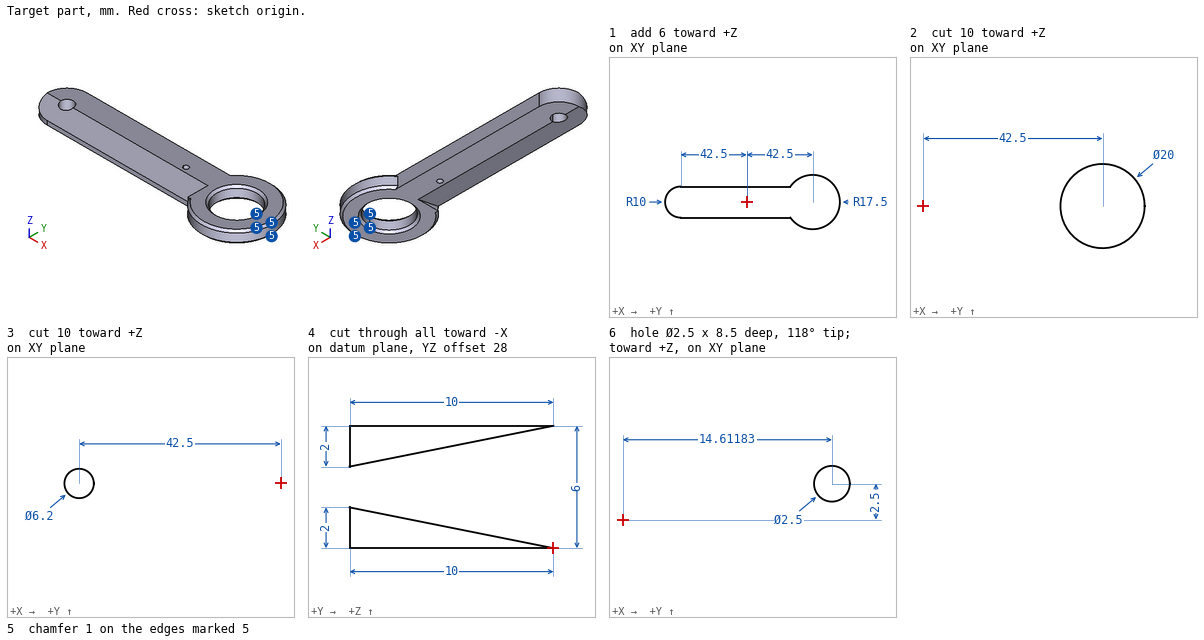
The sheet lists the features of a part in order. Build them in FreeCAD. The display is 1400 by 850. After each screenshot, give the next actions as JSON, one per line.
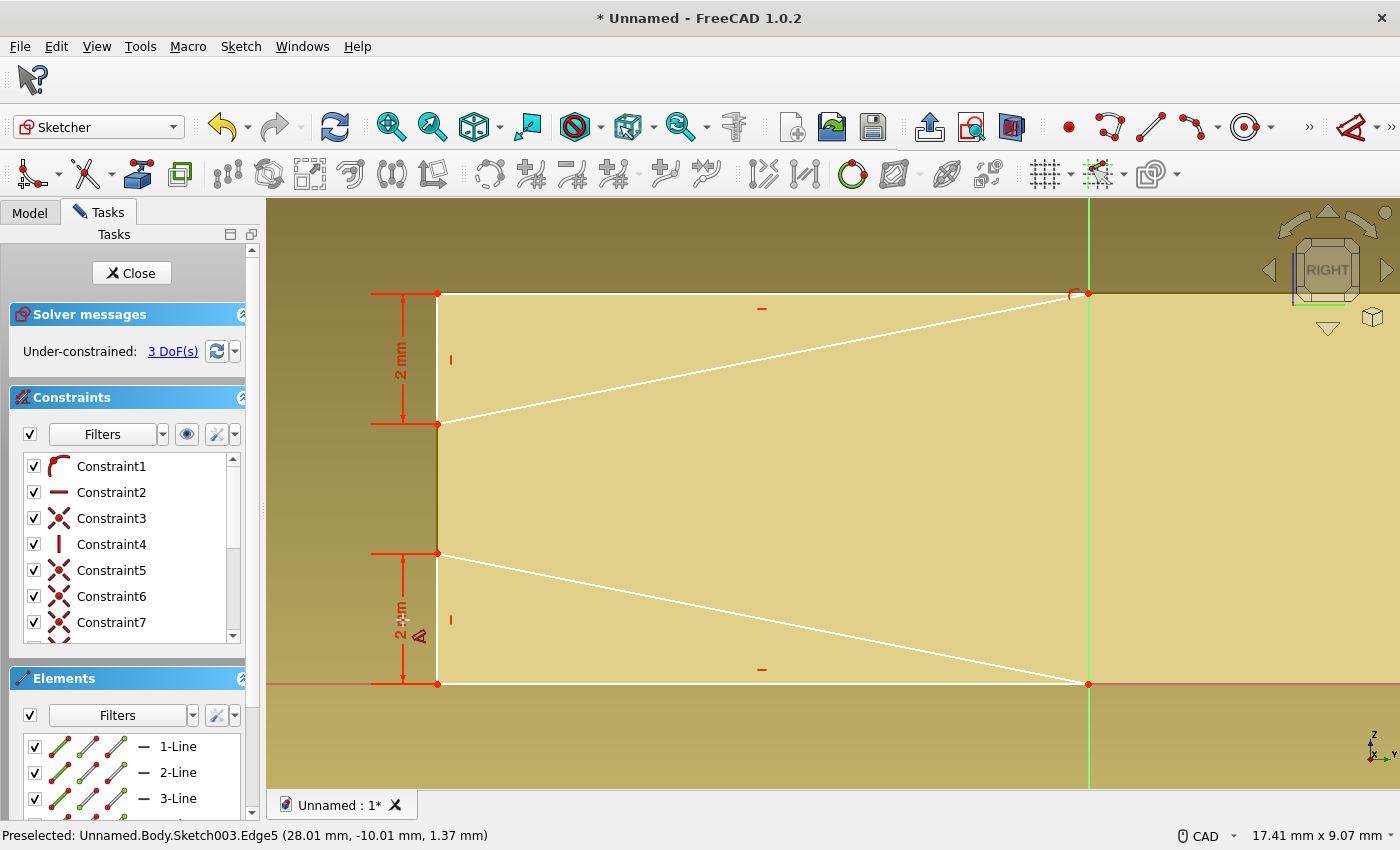
{"action": "left_click", "coordinate": [893, 294]}
{"action": "left_click", "coordinate": [763, 260]}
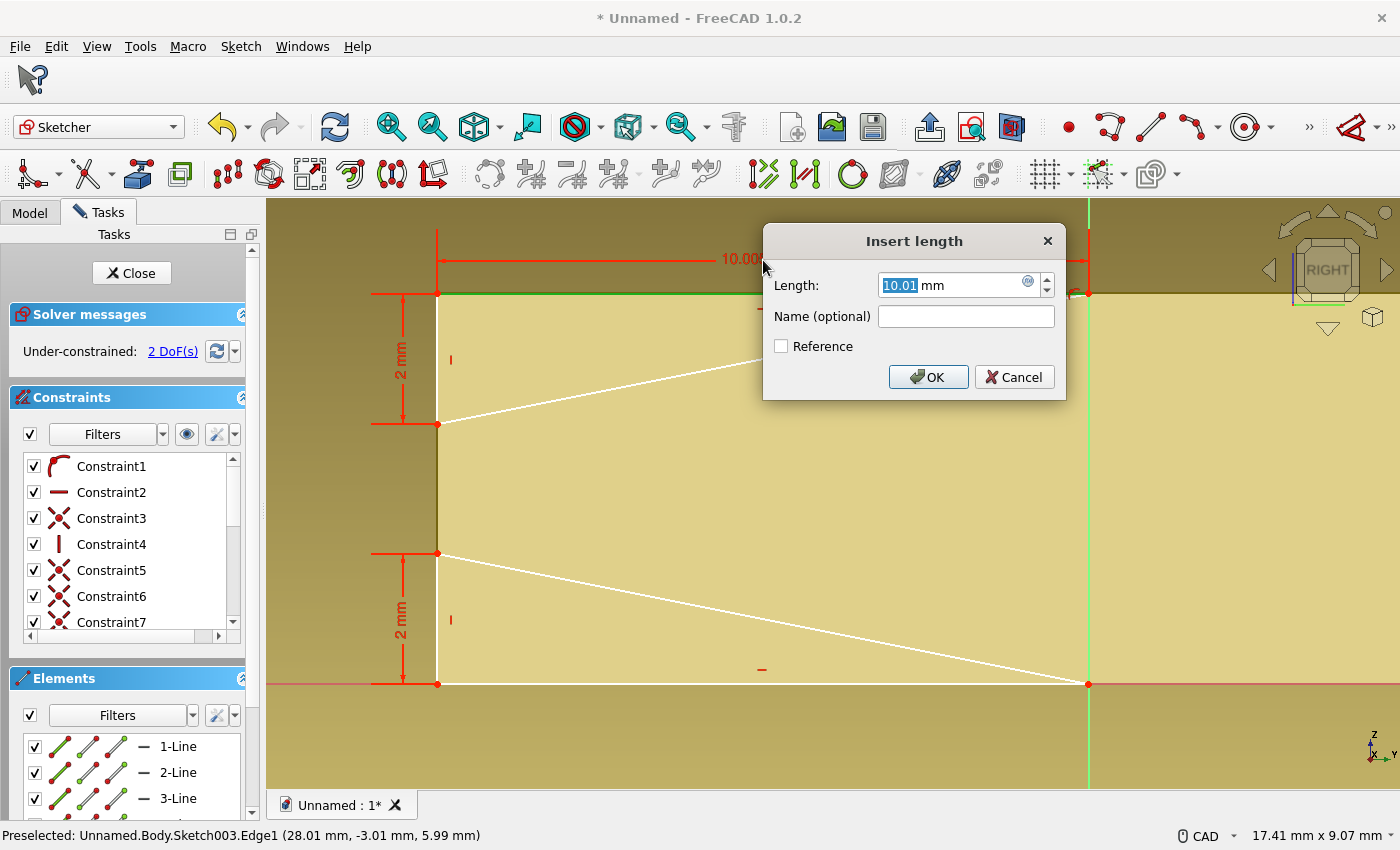
{"action": "type", "text": "10"}
{"action": "key", "text": "Return"}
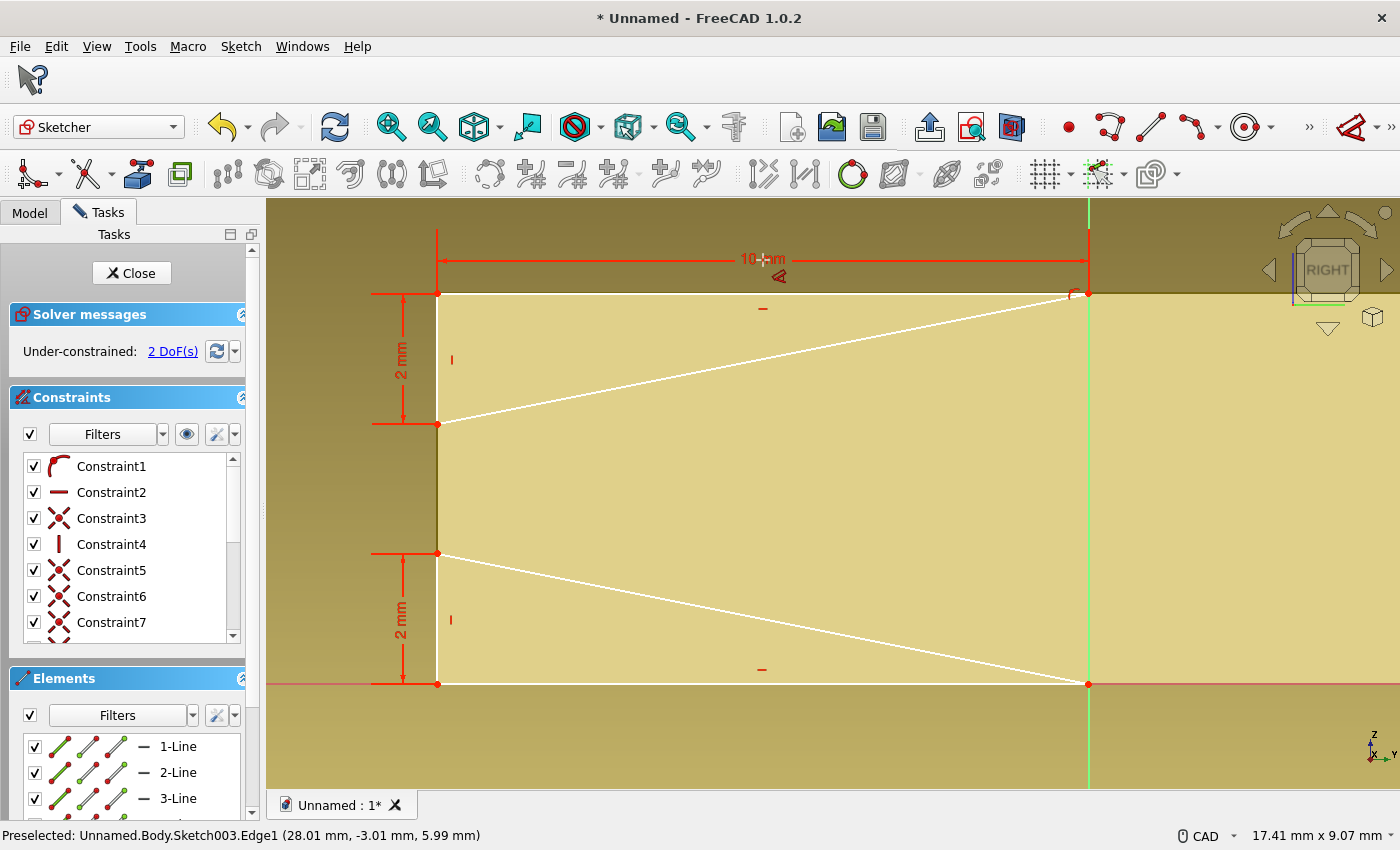
{"action": "left_click", "coordinate": [633, 684]}
{"action": "left_click", "coordinate": [763, 718]}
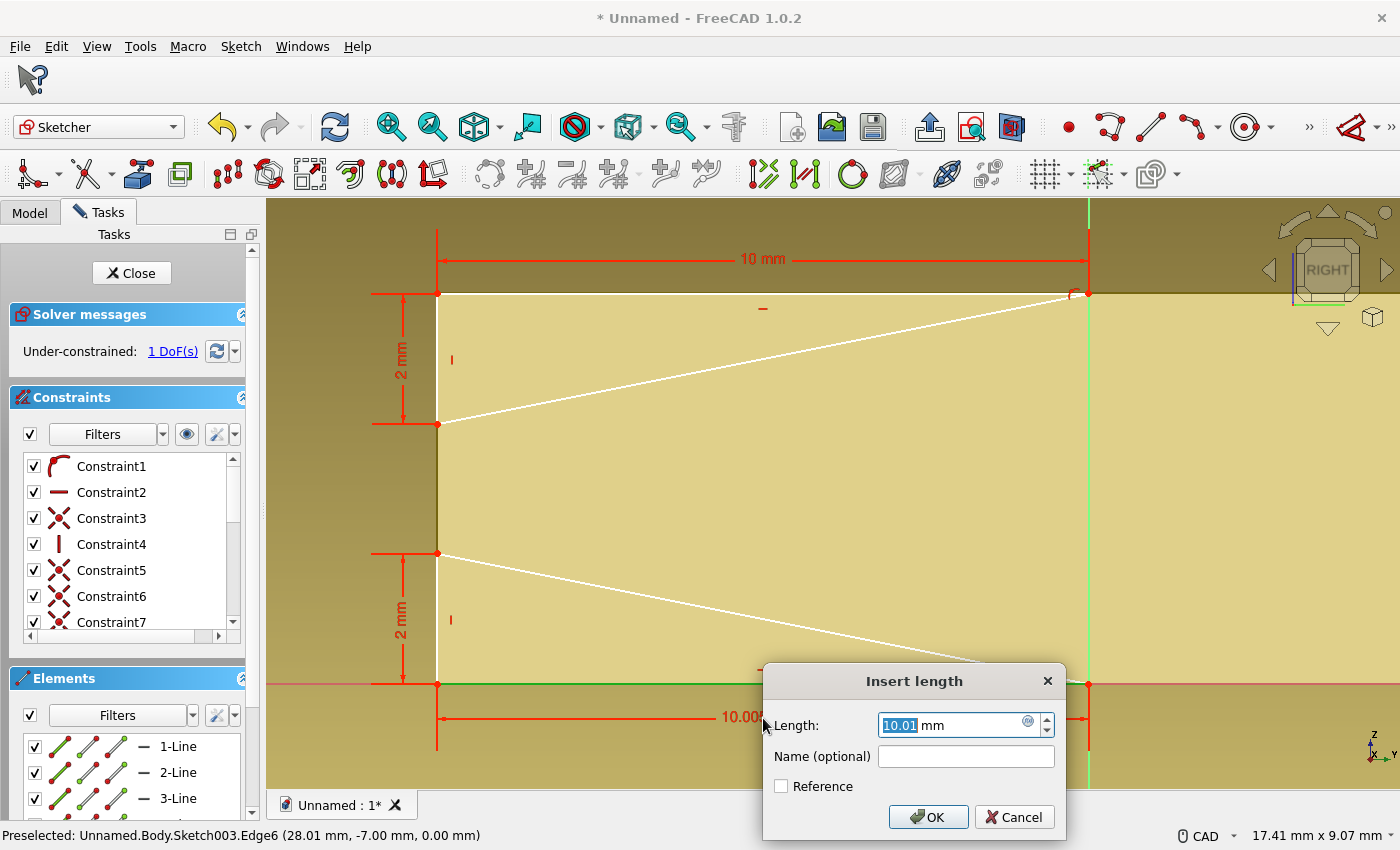
{"action": "type", "text": "10"}
{"action": "key", "text": "Return"}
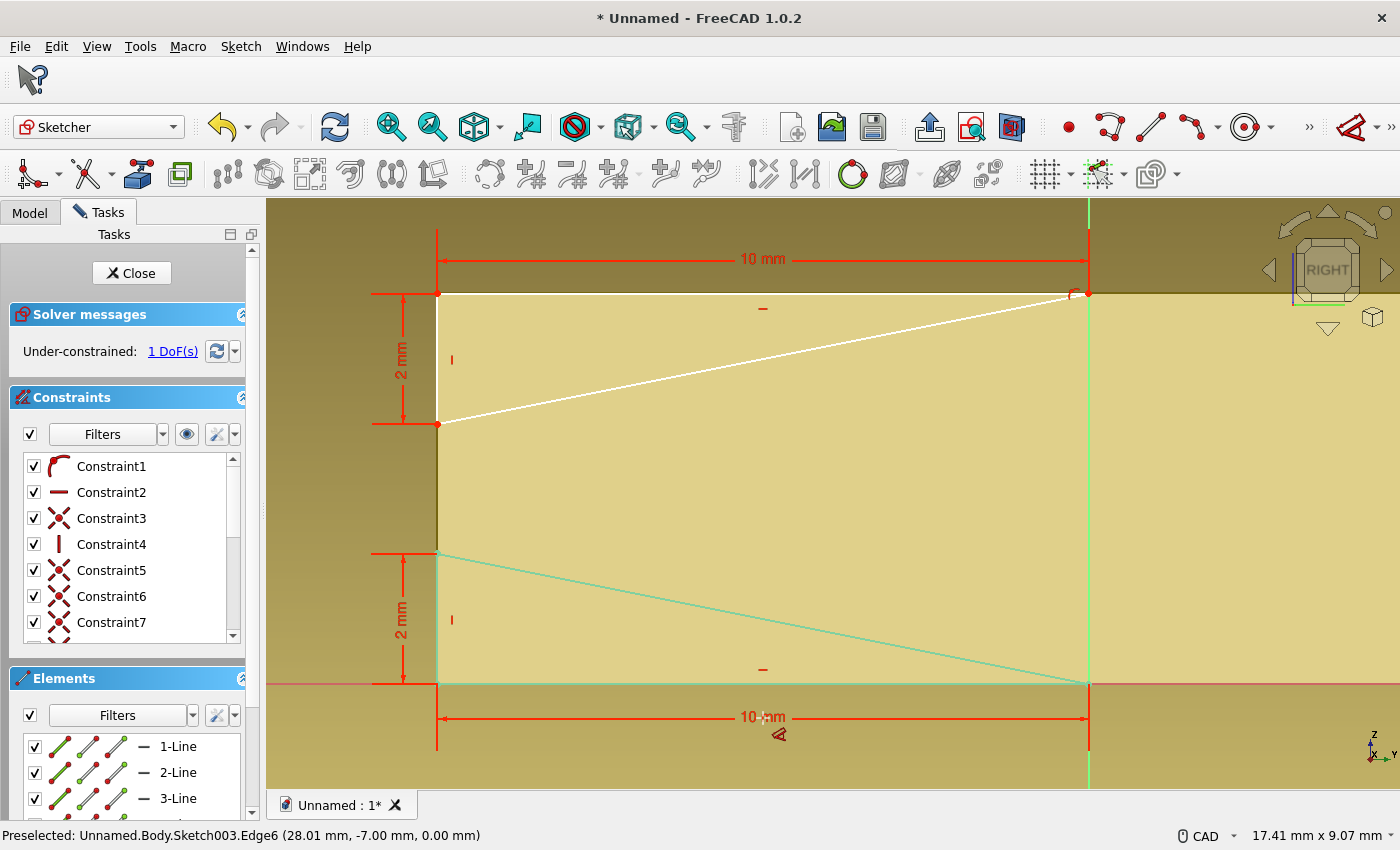
{"action": "left_click", "coordinate": [1089, 294]}
{"action": "left_click", "coordinate": [1123, 489]}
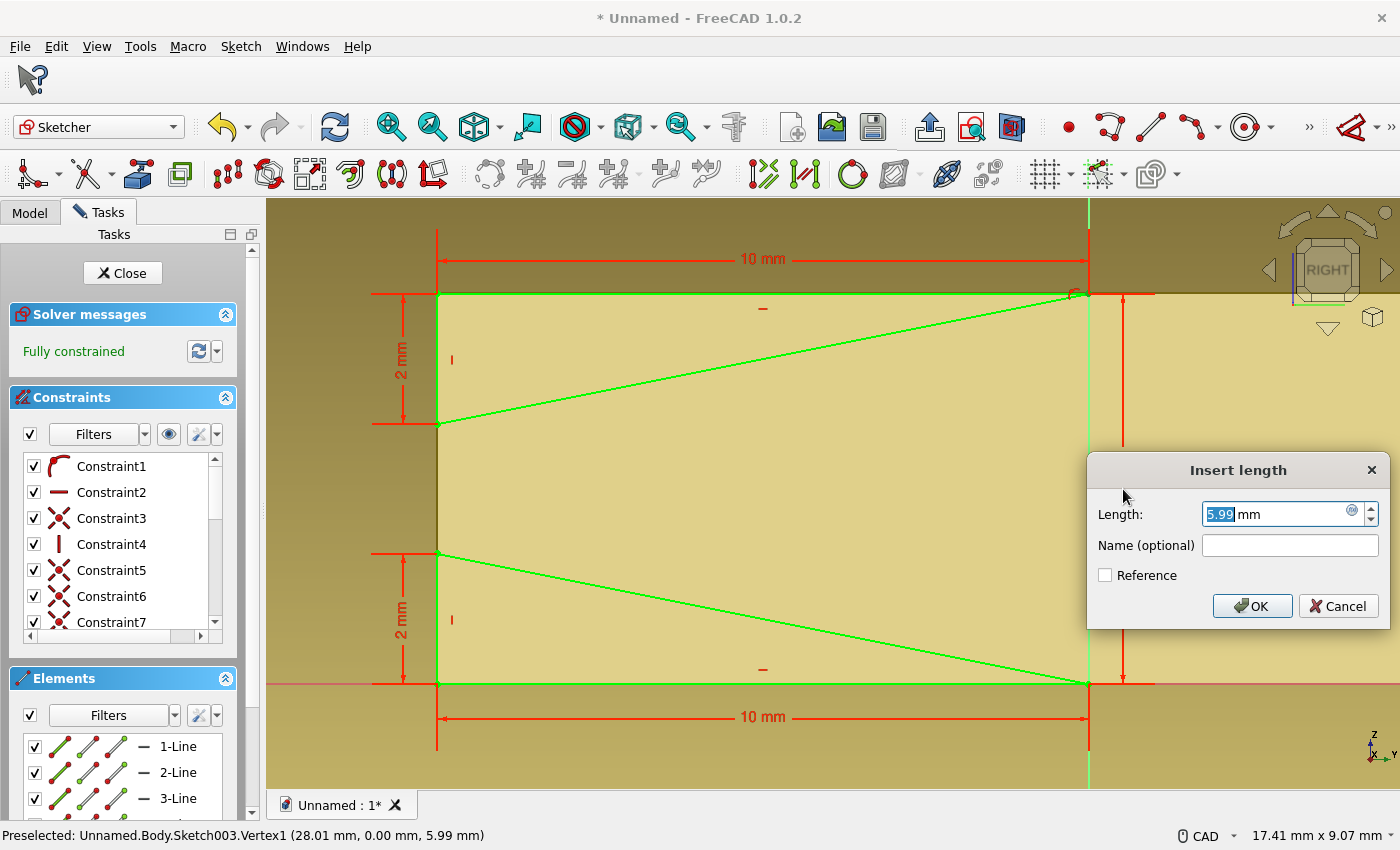
{"action": "type", "text": "6"}
{"action": "key", "text": "Return"}
{"action": "key", "text": "Escape"}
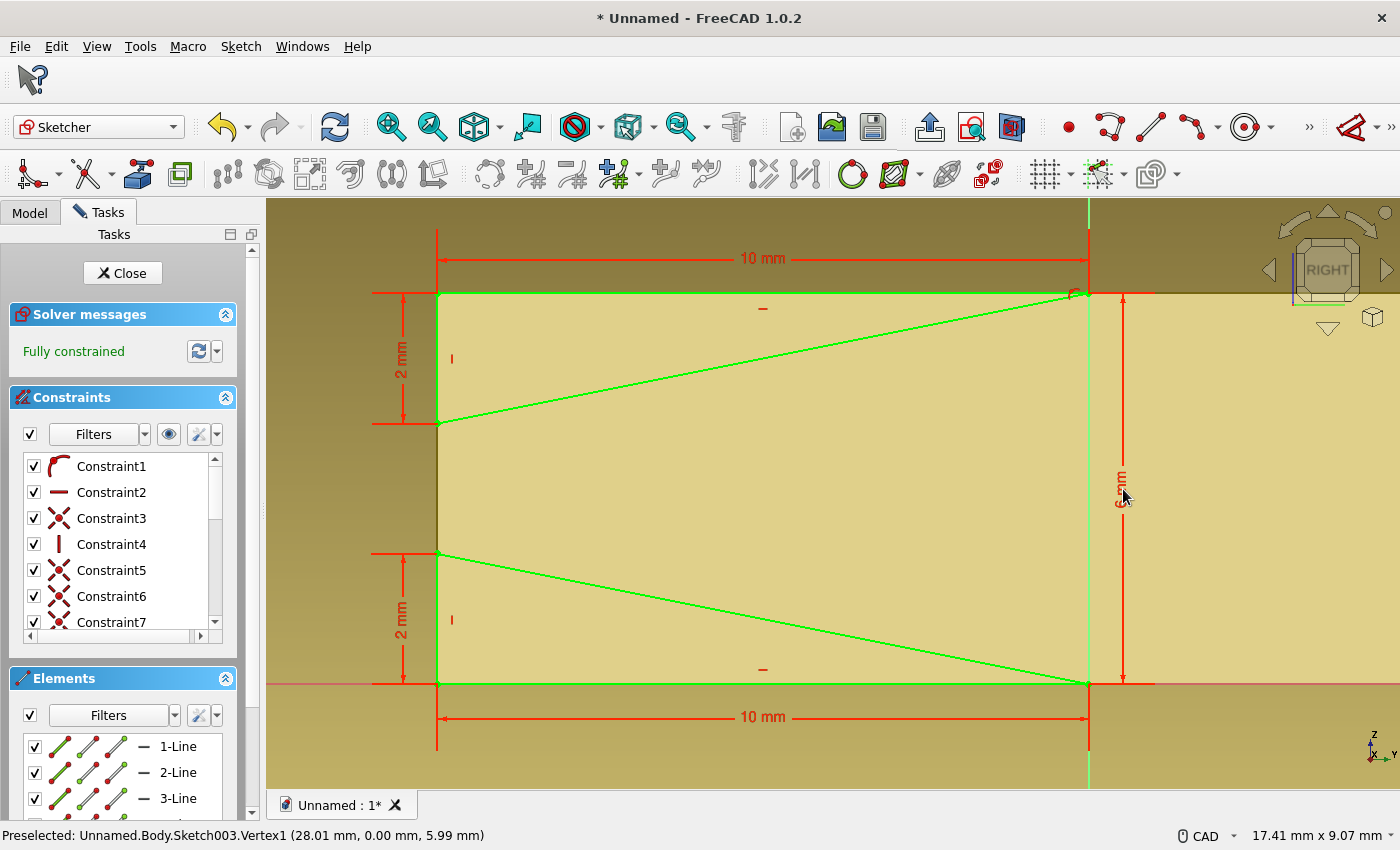
{"action": "left_click", "coordinate": [123, 273]}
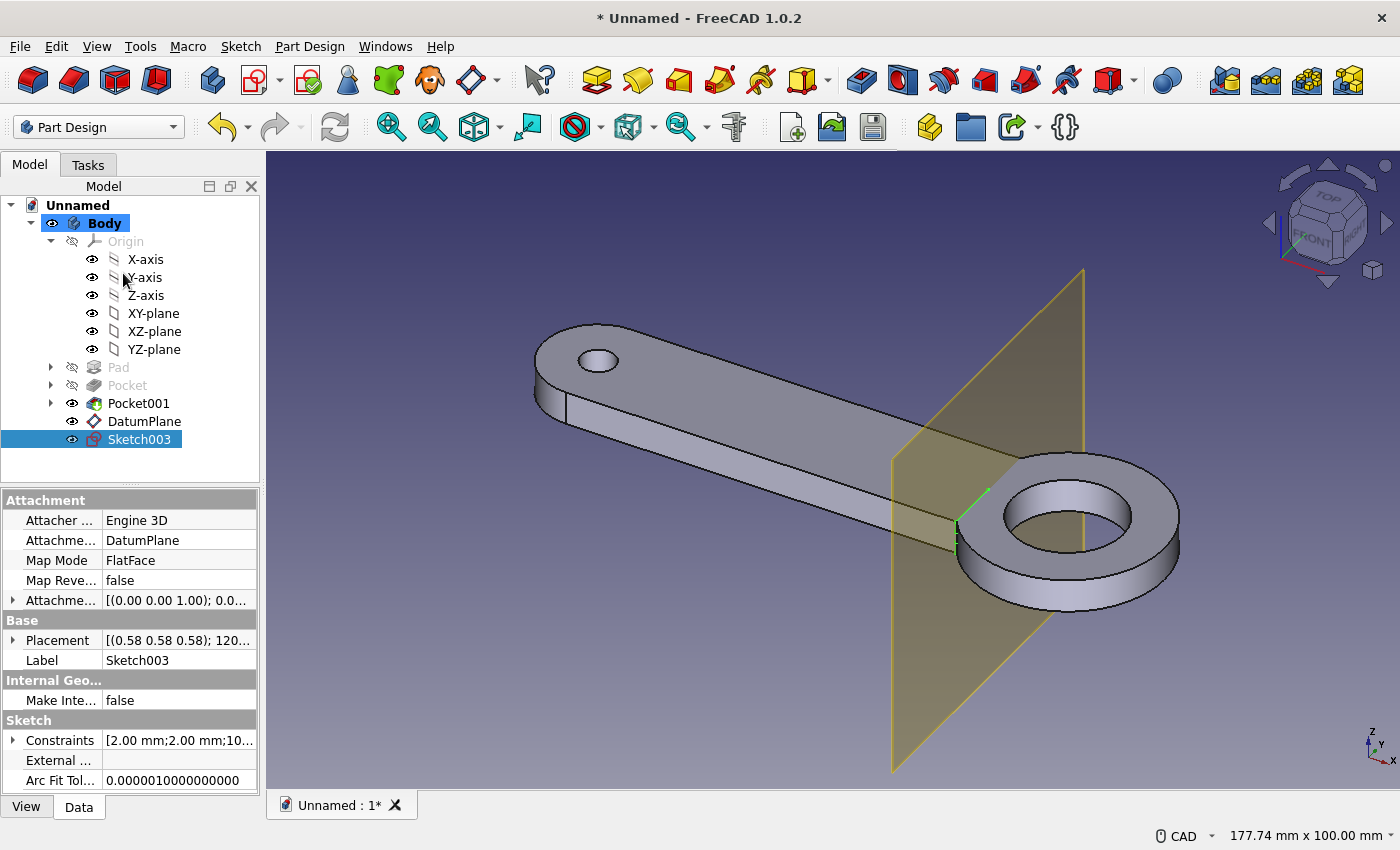
{"action": "left_click", "coordinate": [862, 80]}